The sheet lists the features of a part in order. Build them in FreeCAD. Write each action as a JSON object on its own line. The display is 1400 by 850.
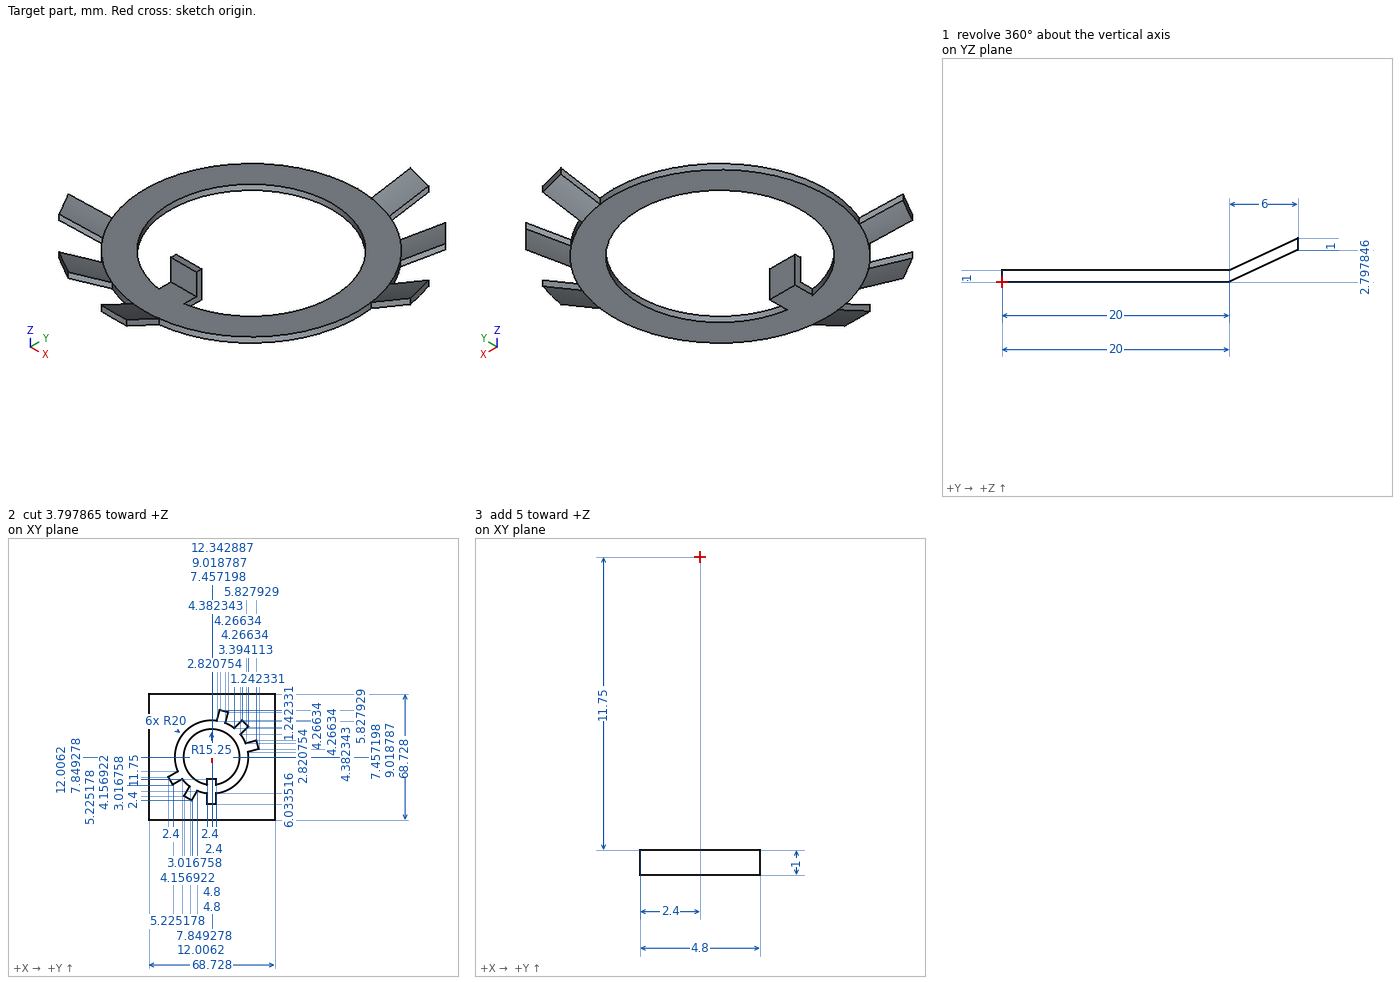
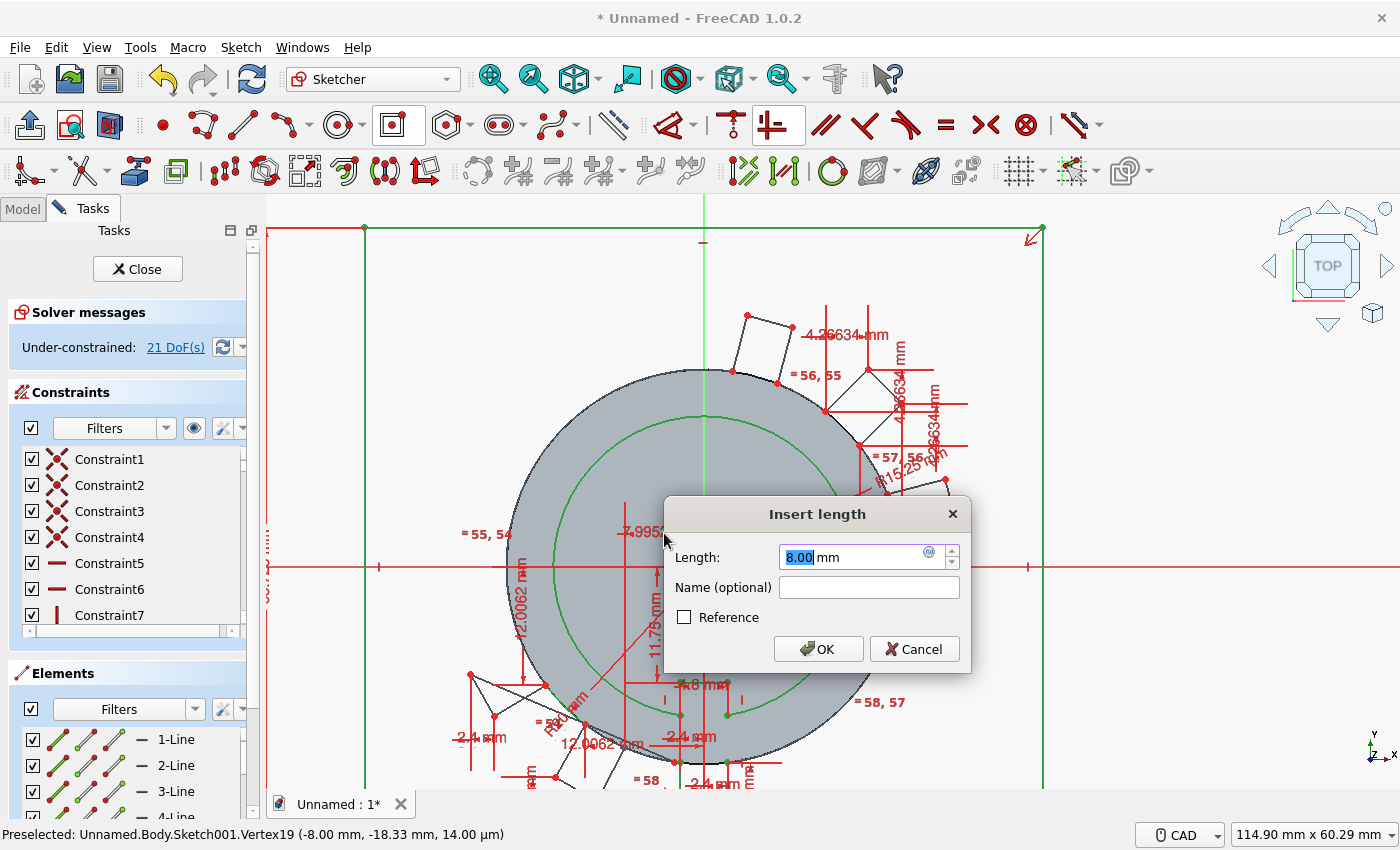
{"action": "type", "text": "7.849278"}
{"action": "key", "text": "Return"}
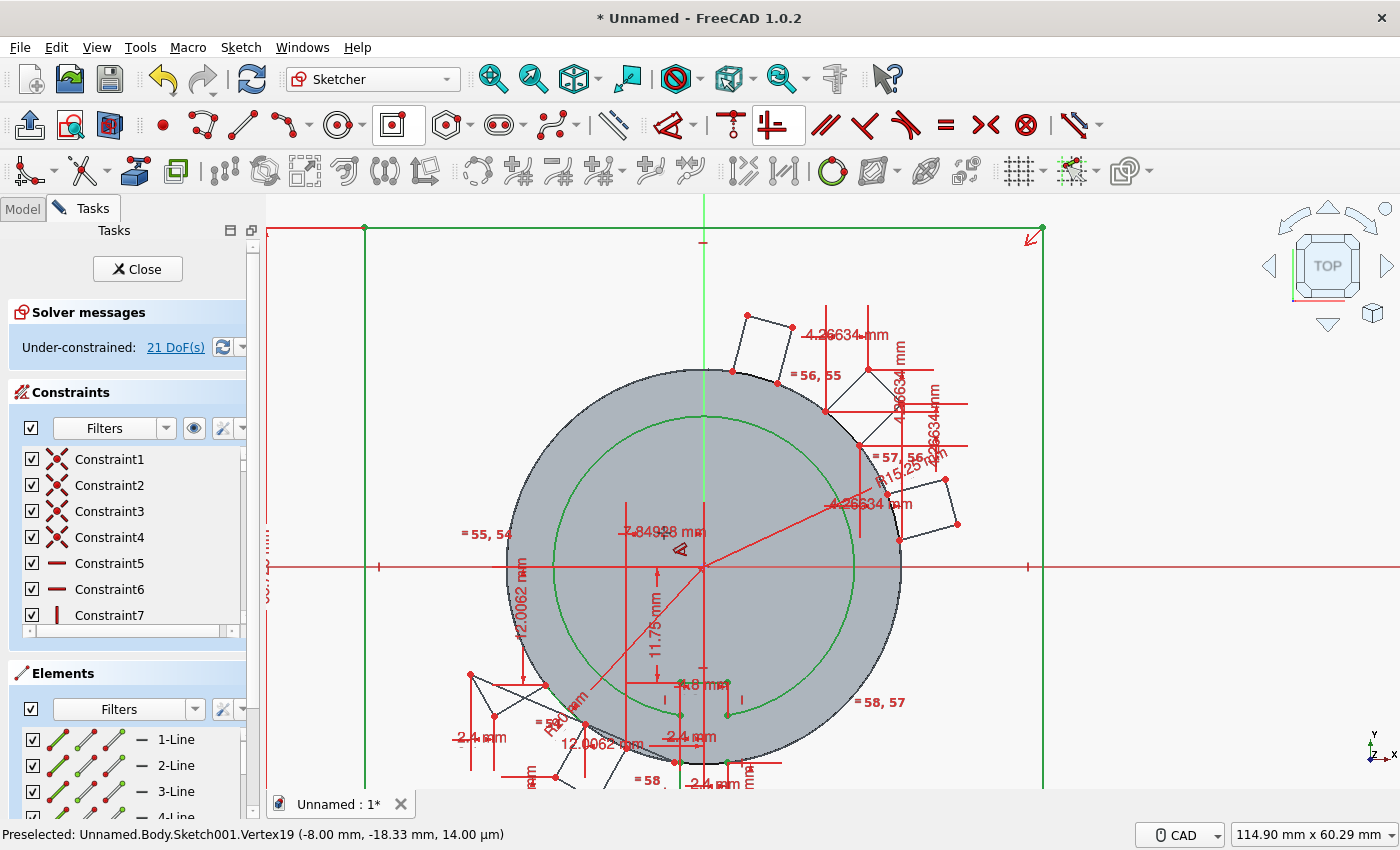
{"action": "scroll", "coordinate": [838, 400], "scroll_direction": "down", "scroll_amount": 3}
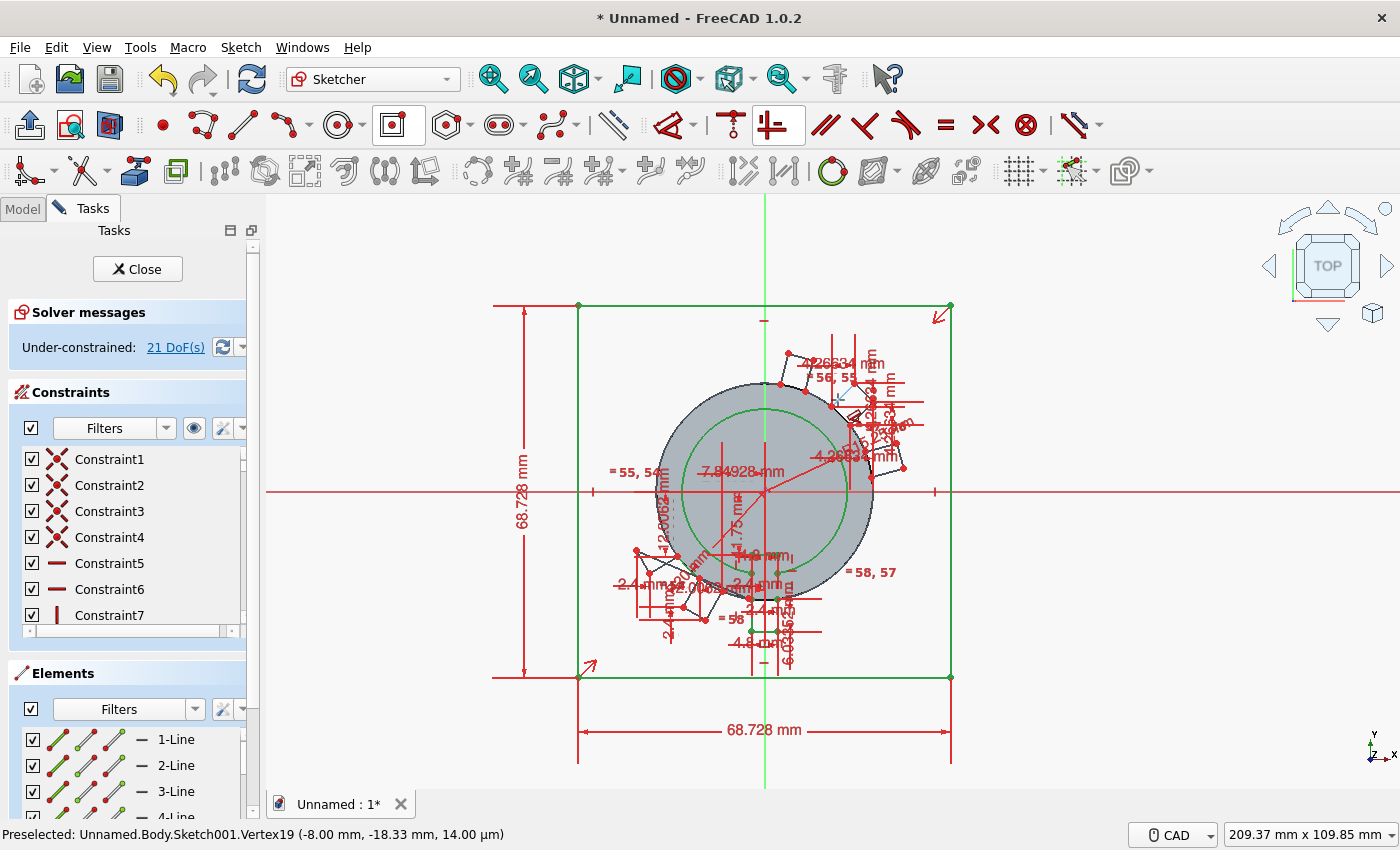
{"action": "scroll", "coordinate": [749, 599], "scroll_direction": "up", "scroll_amount": 7}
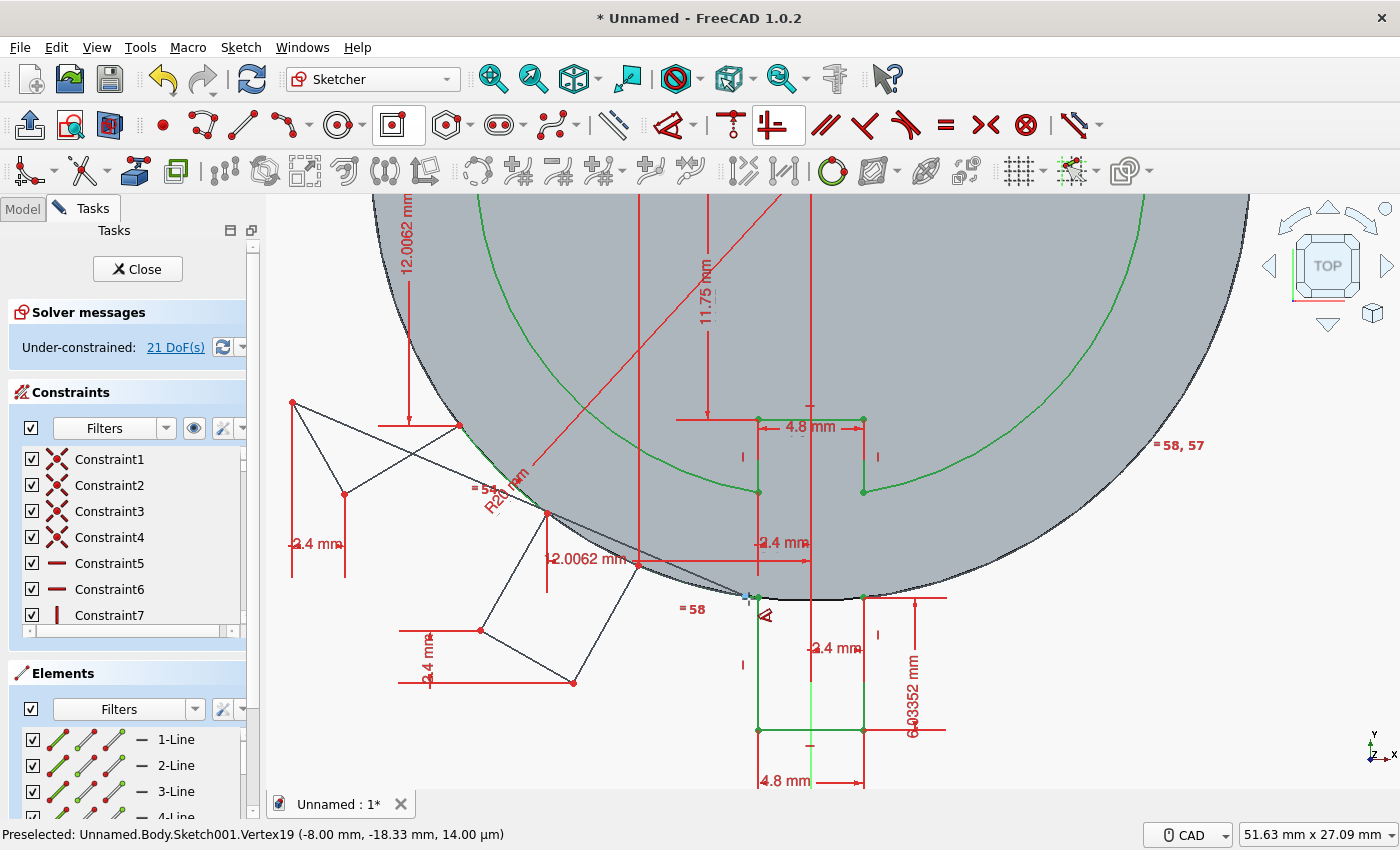
{"action": "left_click", "coordinate": [746, 596]}
{"action": "left_click", "coordinate": [712, 409]}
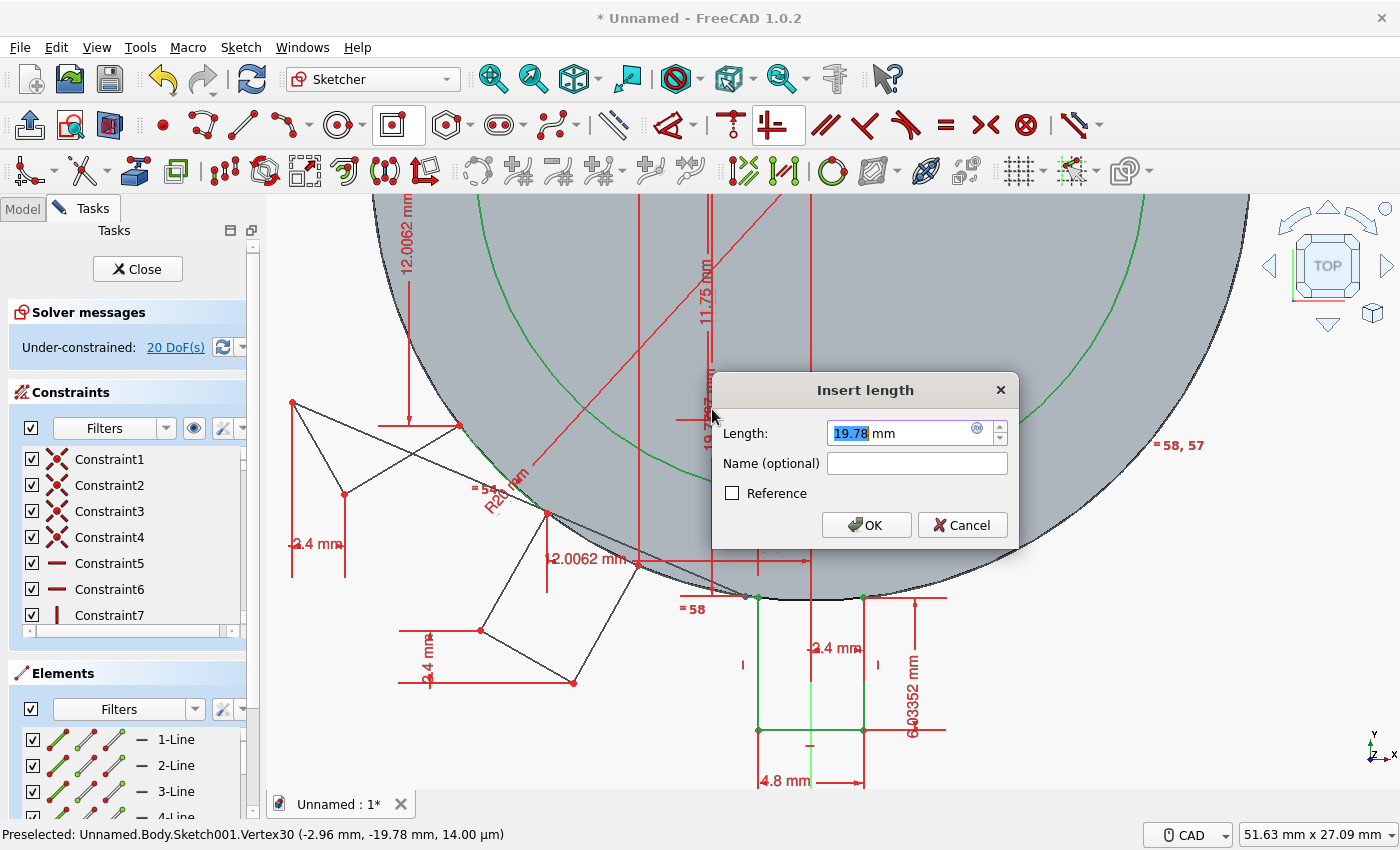
{"action": "type", "text": "7.849278"}
{"action": "key", "text": "Return"}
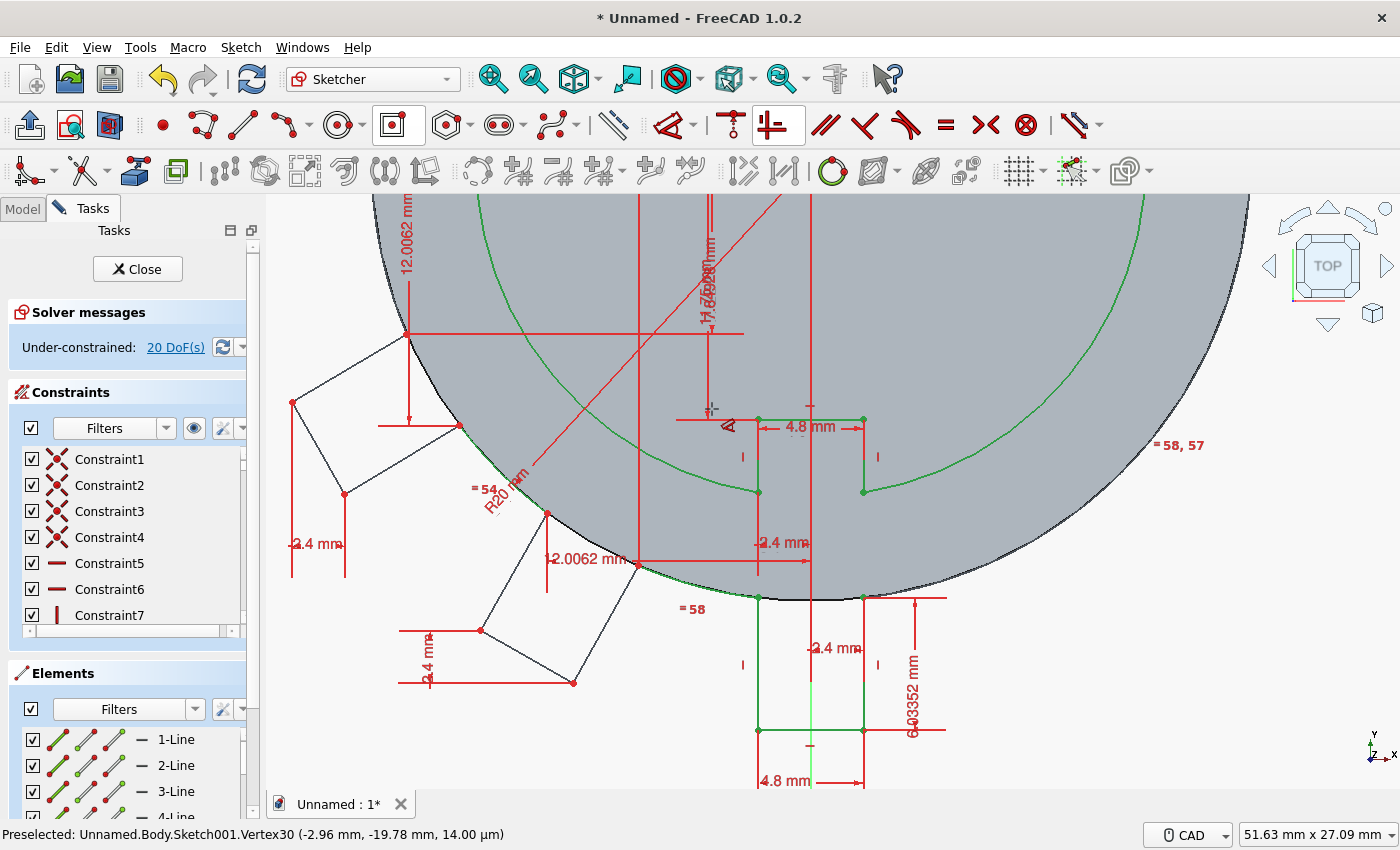
{"action": "scroll", "coordinate": [749, 599], "scroll_direction": "down", "scroll_amount": 7}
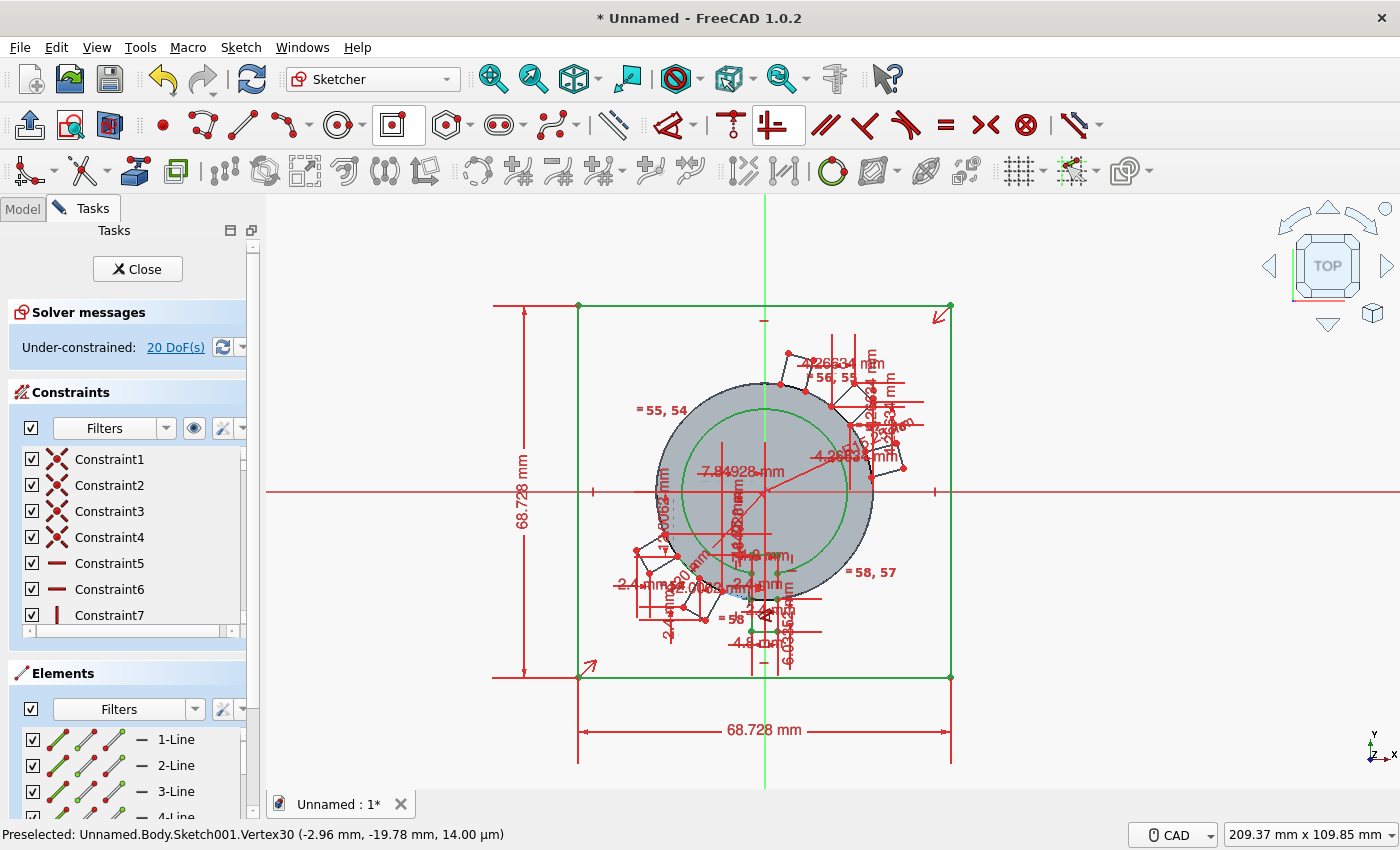
{"action": "scroll", "coordinate": [781, 385], "scroll_direction": "up", "scroll_amount": 5}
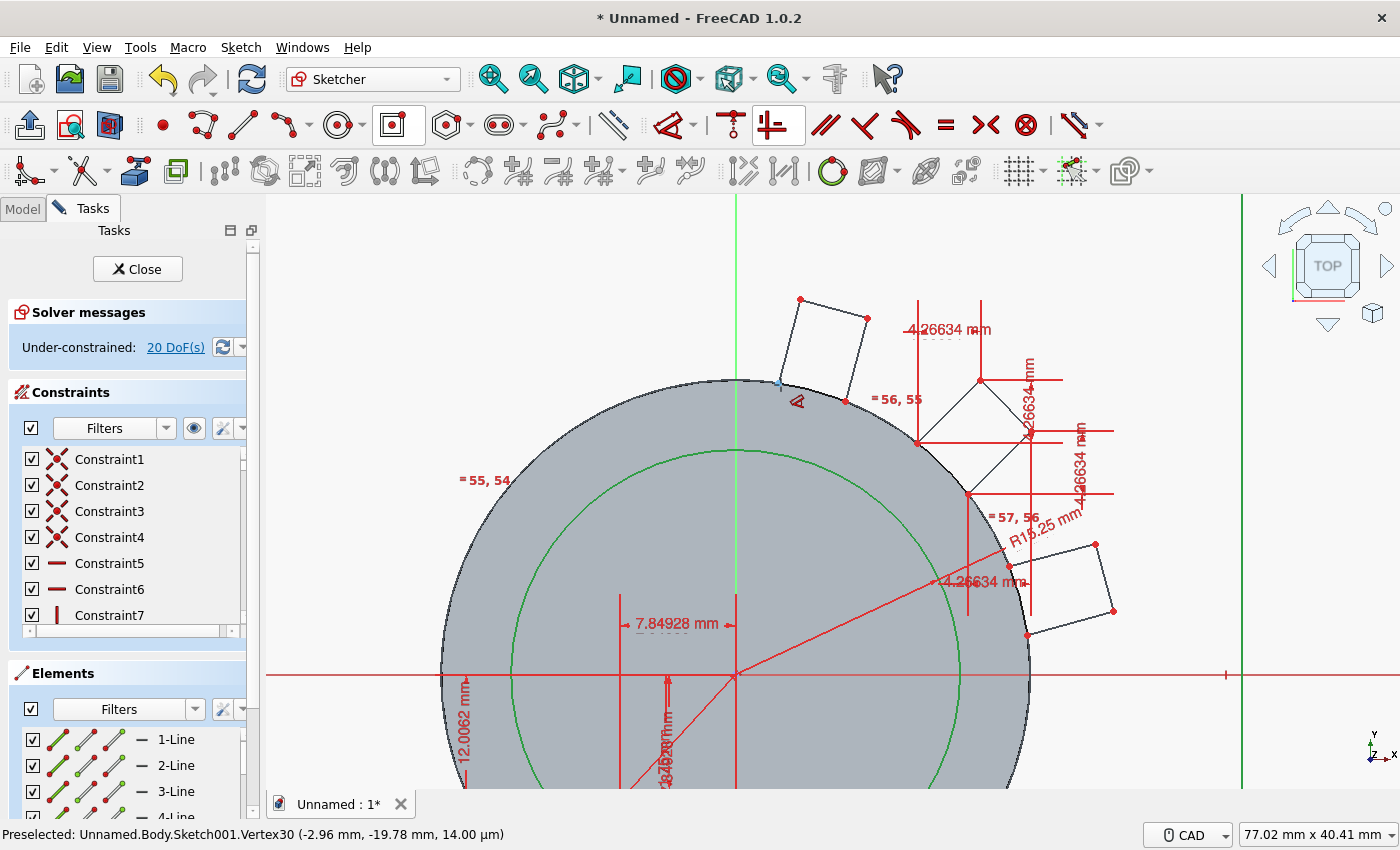
{"action": "left_click", "coordinate": [779, 383]}
{"action": "left_click", "coordinate": [757, 349]}